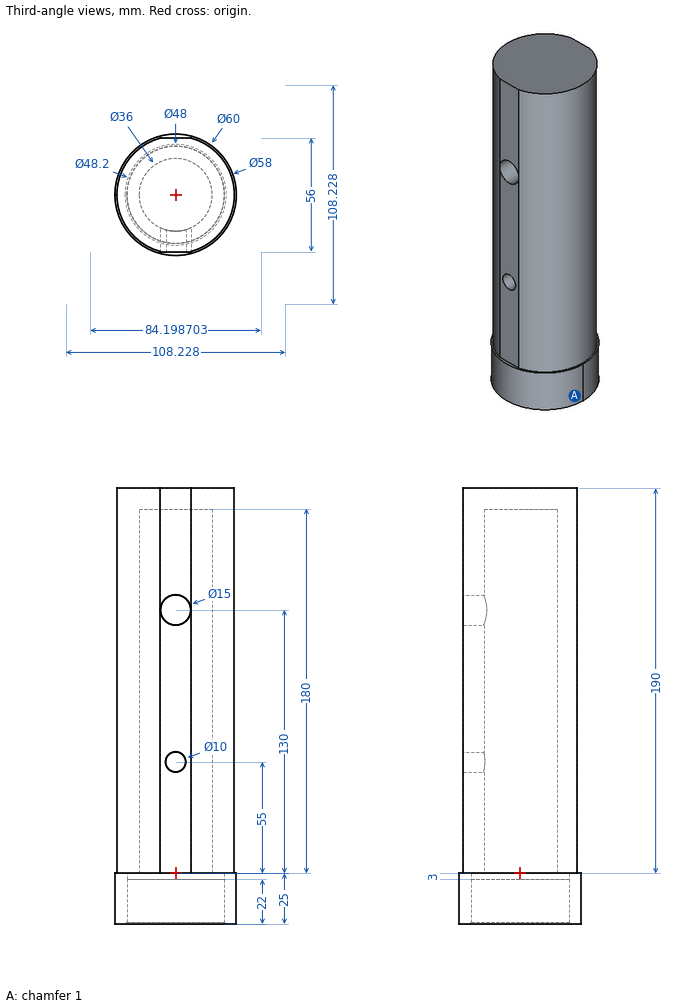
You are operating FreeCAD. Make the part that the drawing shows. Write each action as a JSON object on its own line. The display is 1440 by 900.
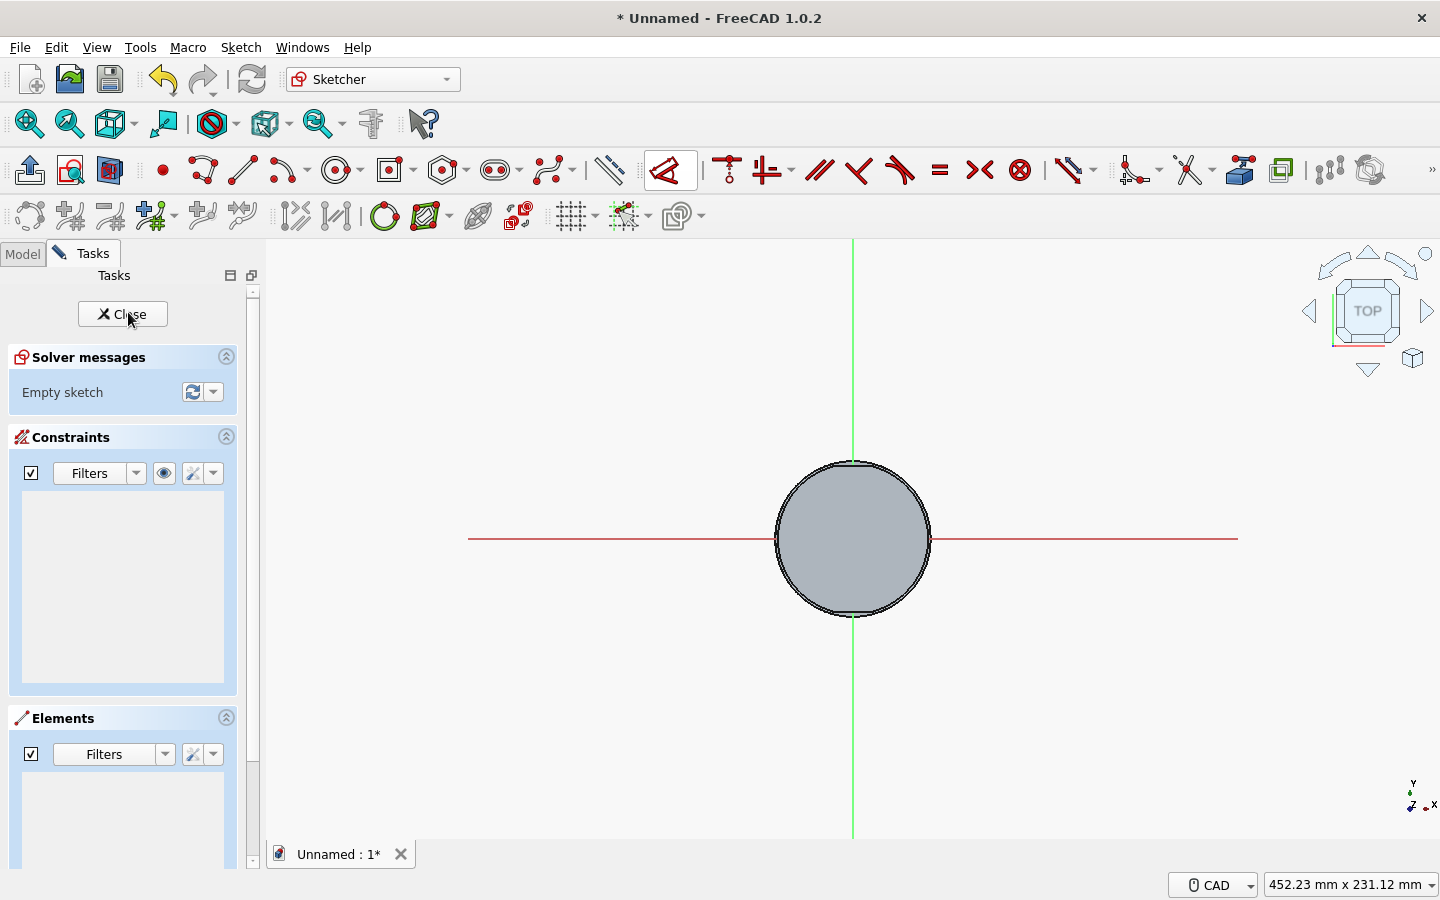
{"action": "left_click", "coordinate": [110, 170]}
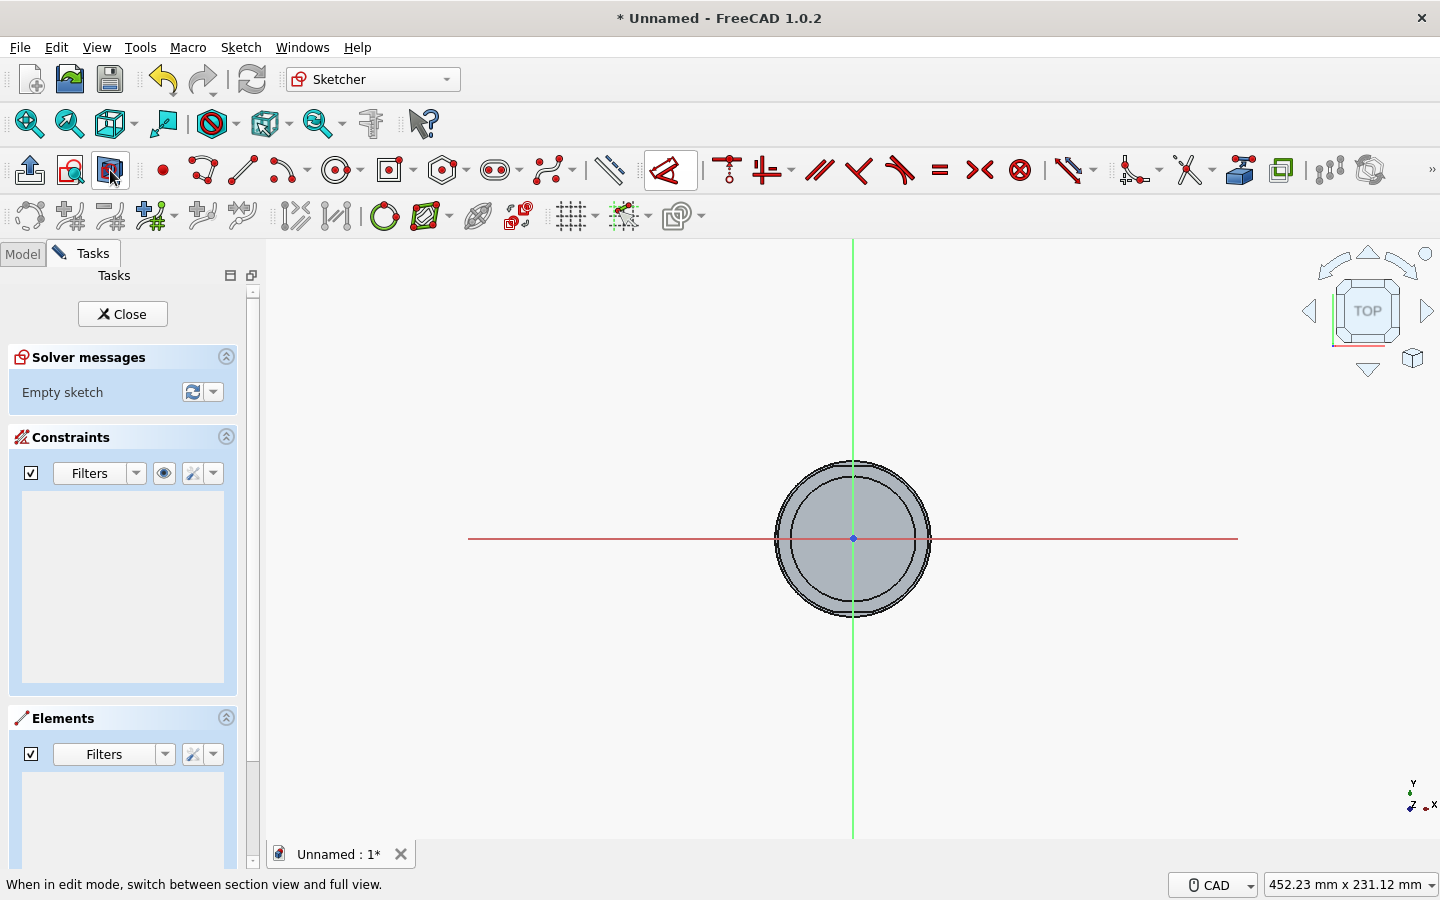
{"action": "scroll", "coordinate": [875, 539], "scroll_direction": "up", "scroll_amount": 7}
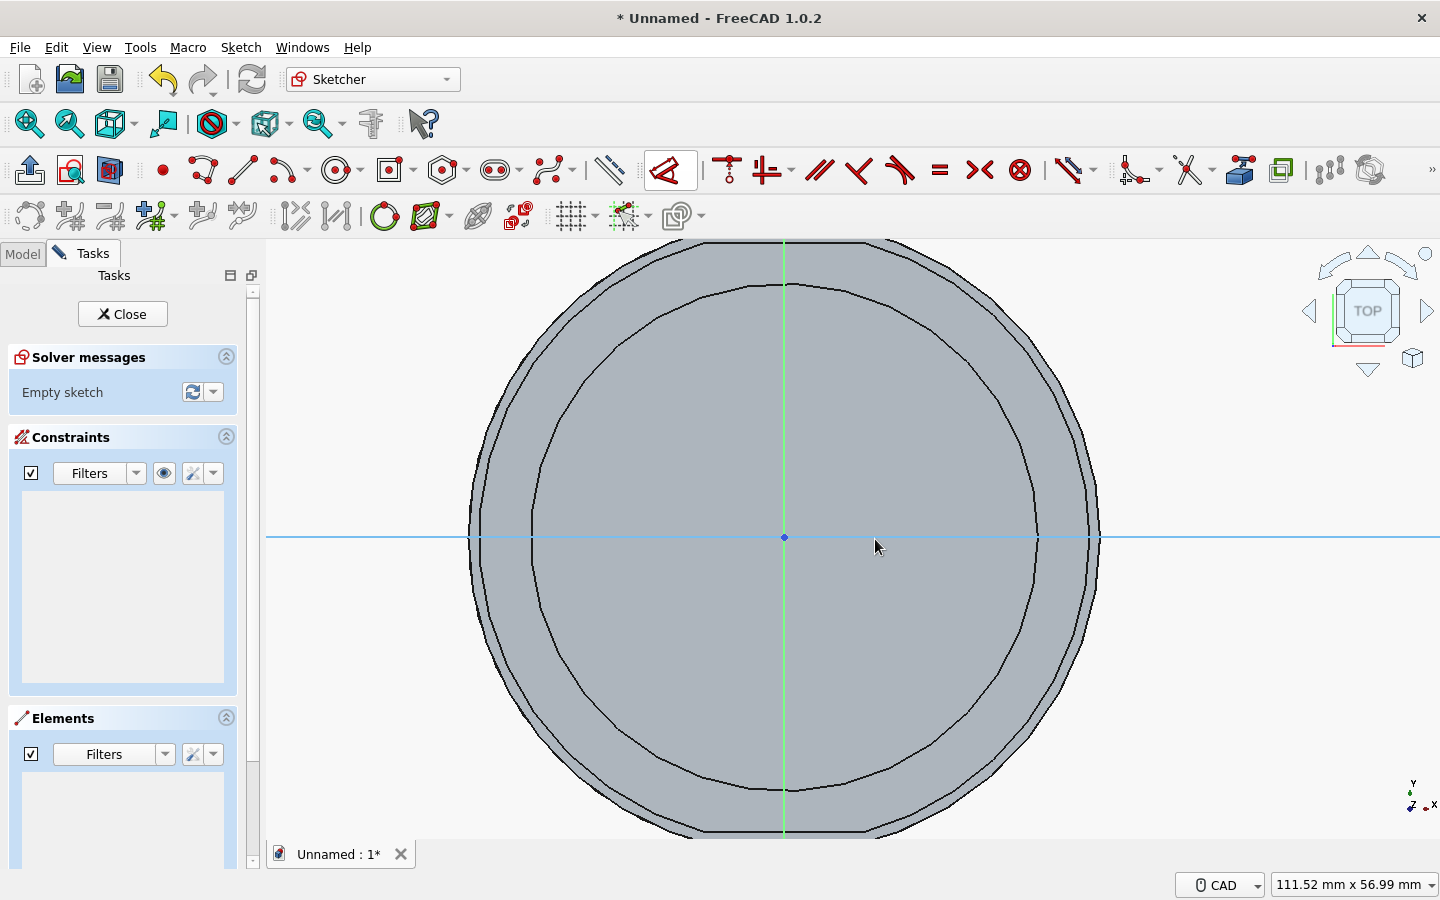
{"action": "left_click", "coordinate": [336, 170]}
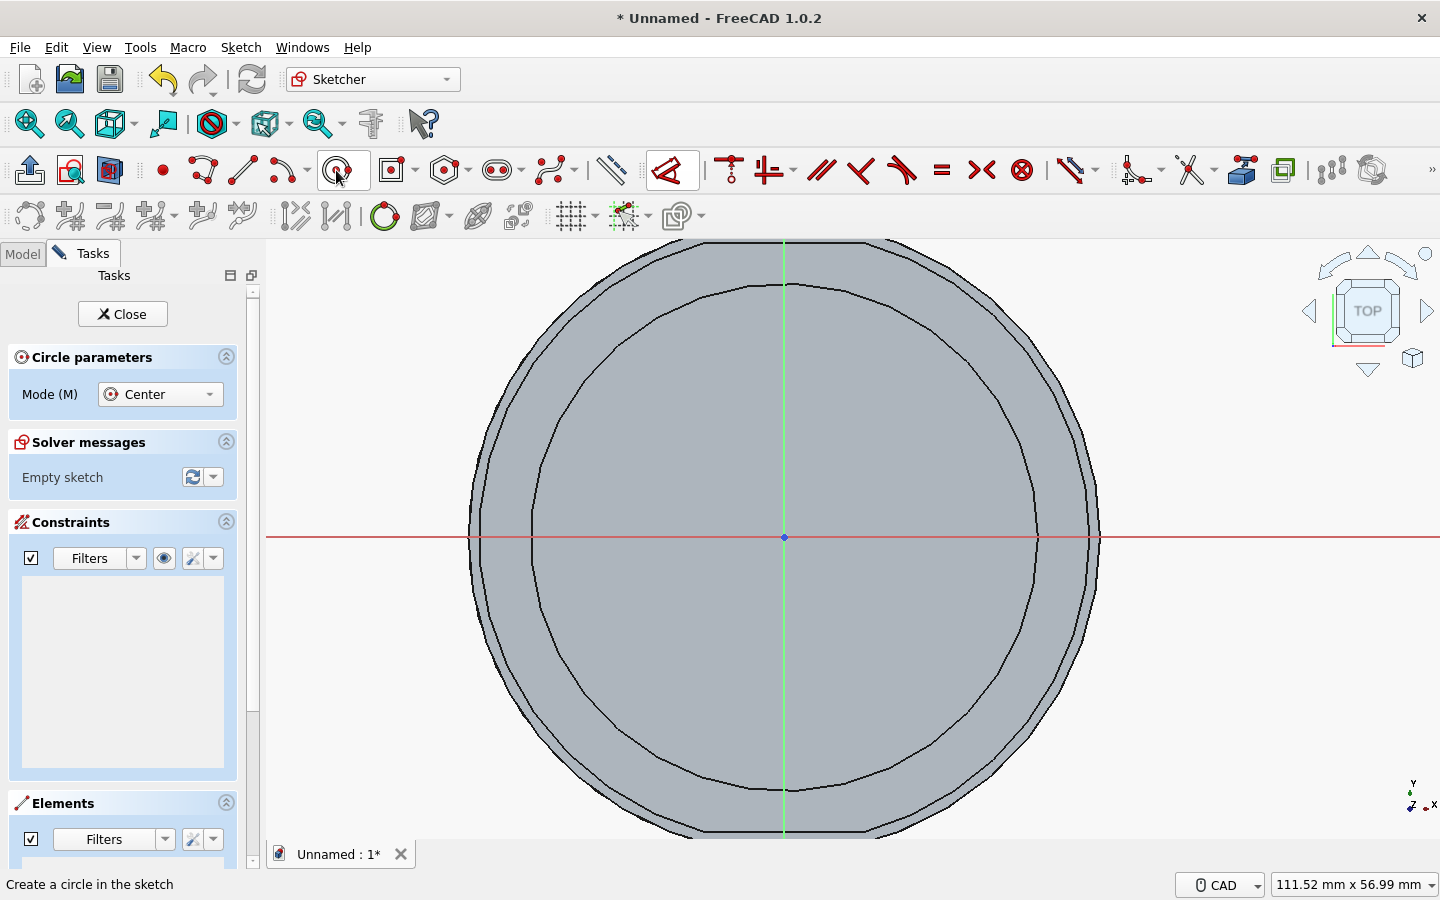
{"action": "left_click", "coordinate": [784, 537]}
{"action": "left_click", "coordinate": [918, 403]}
{"action": "key", "text": "Escape"}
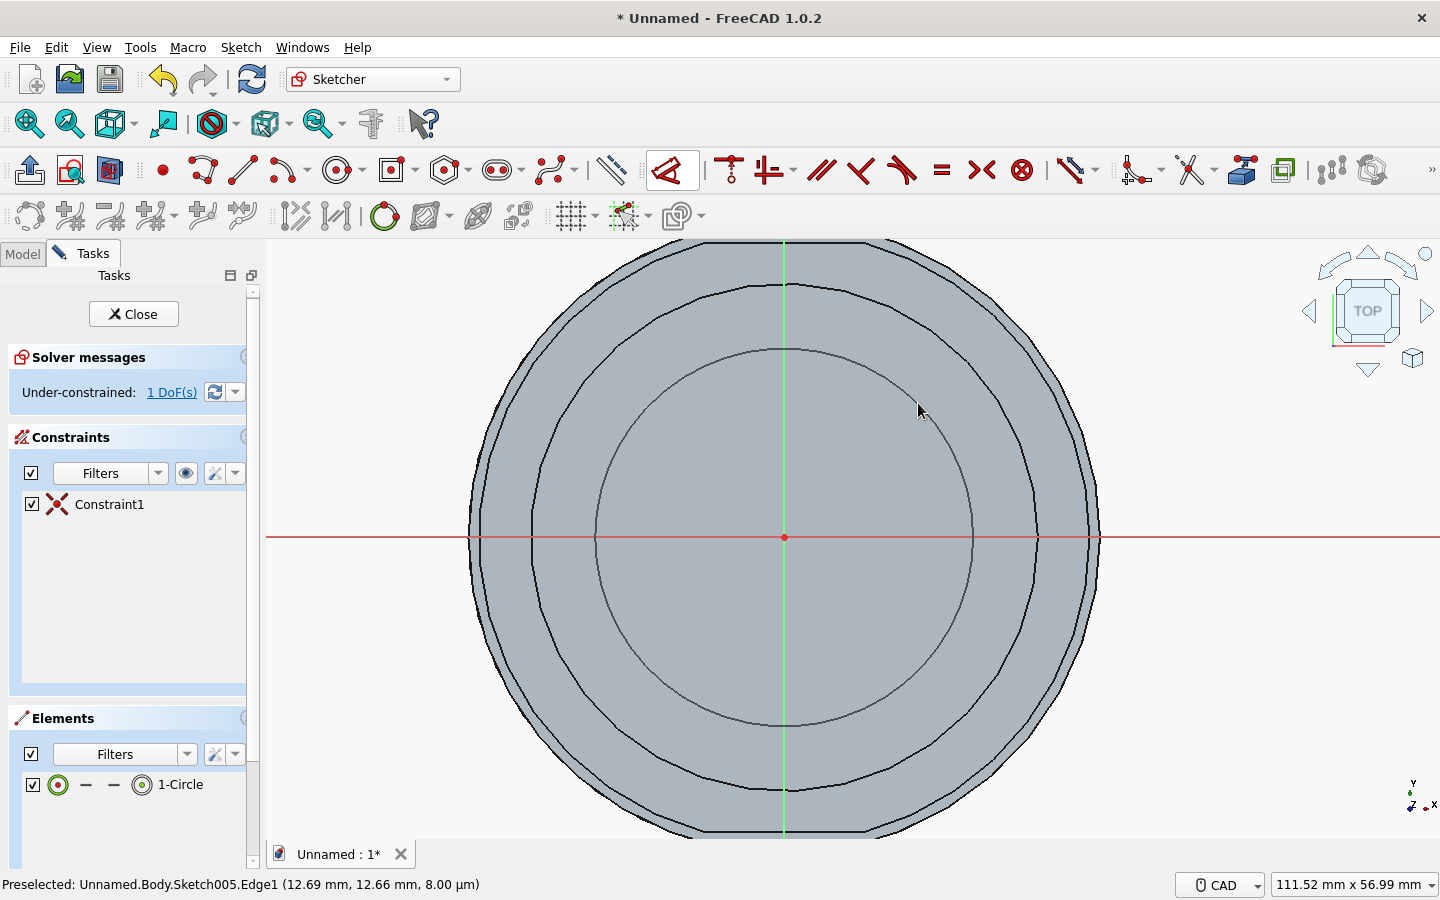
{"action": "left_click", "coordinate": [917, 403]}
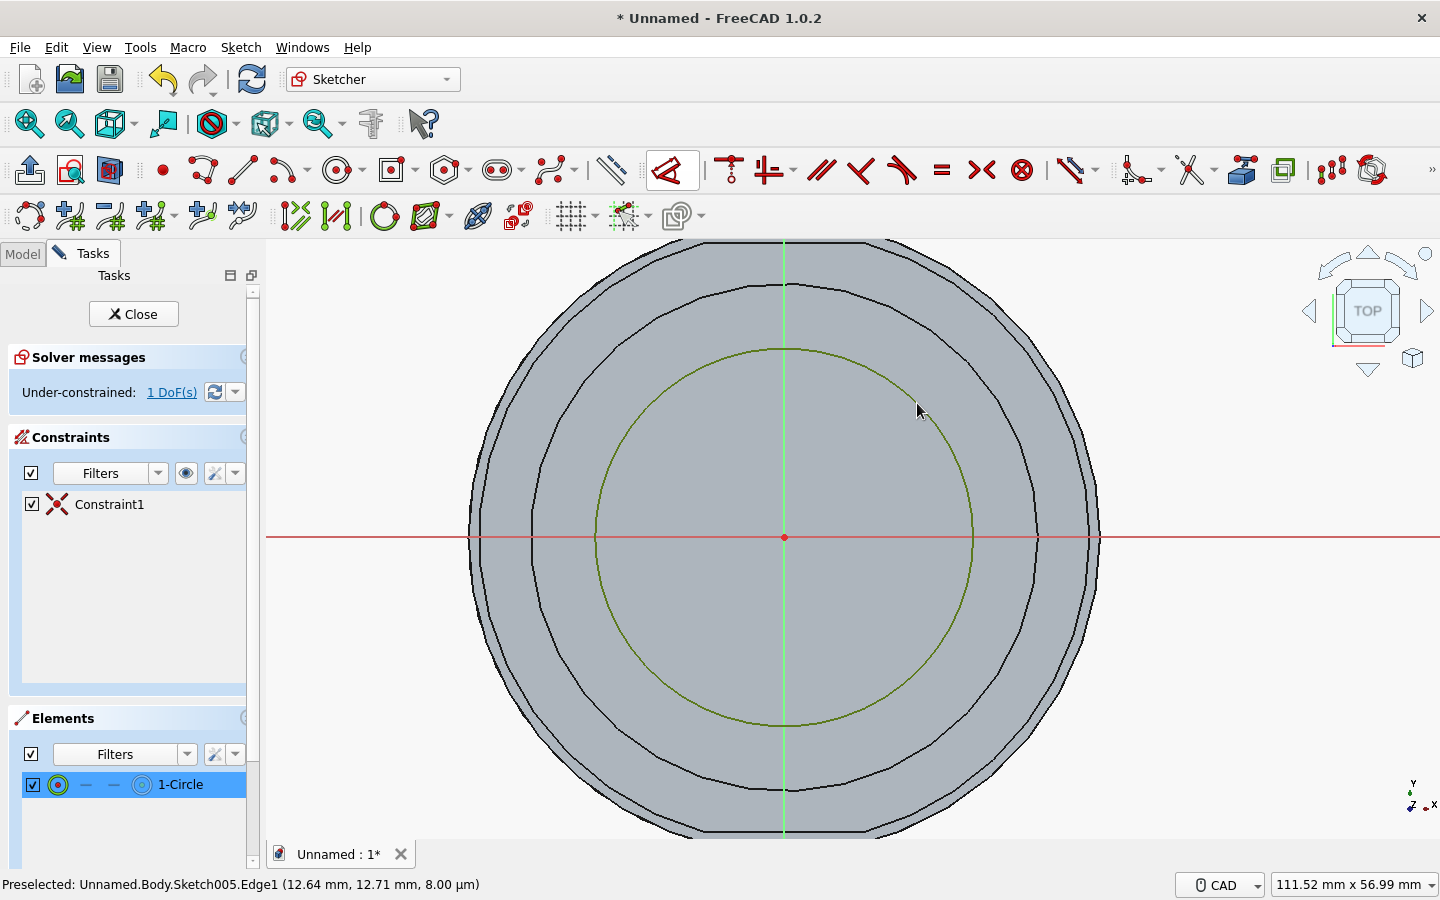
{"action": "key", "text": "k o"}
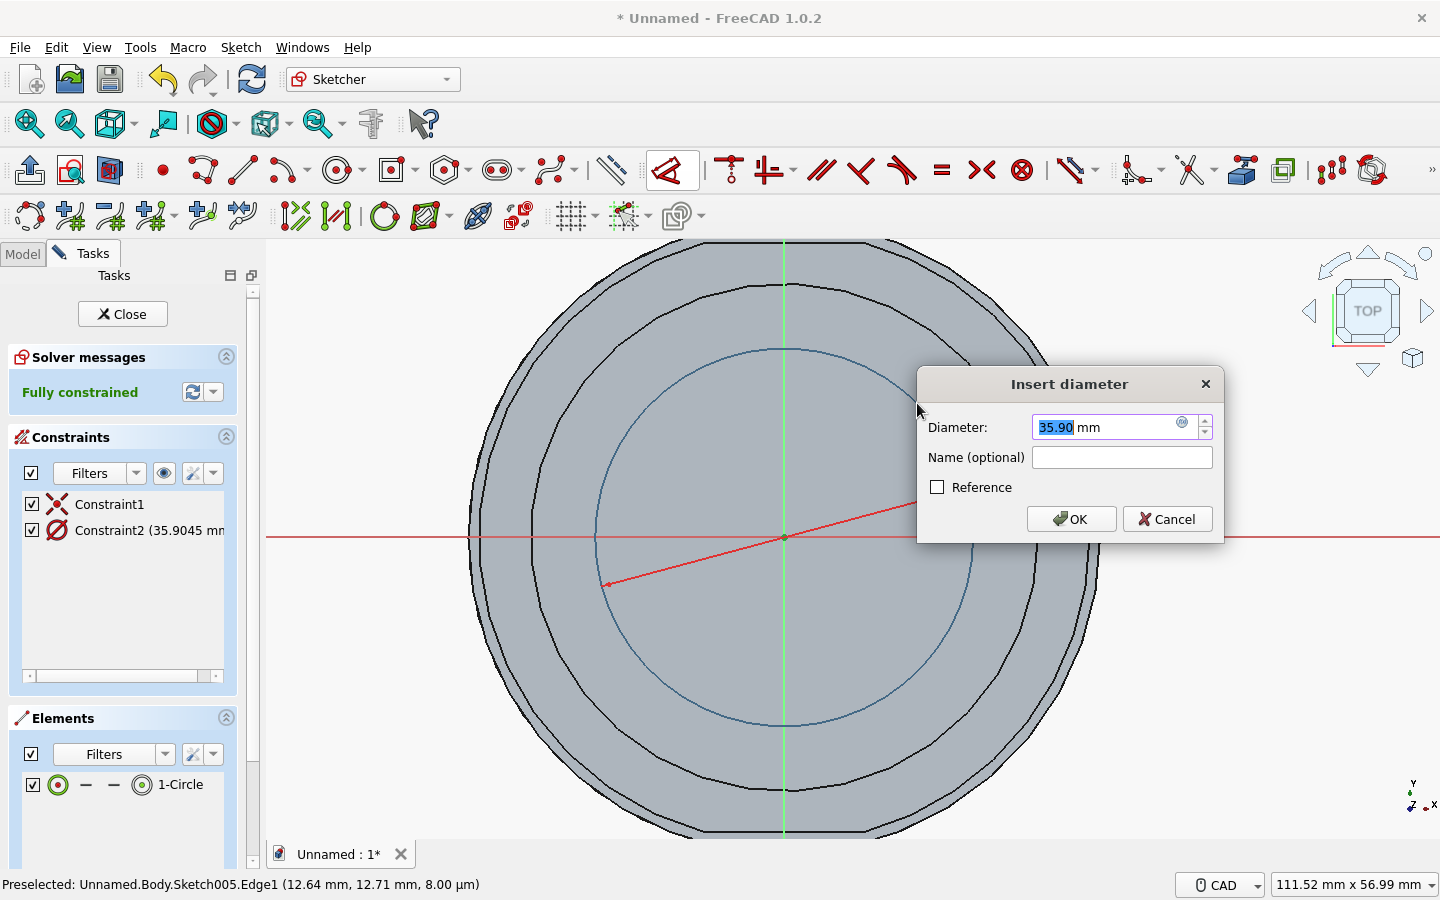
{"action": "type", "text": "36"}
{"action": "key", "text": "Return"}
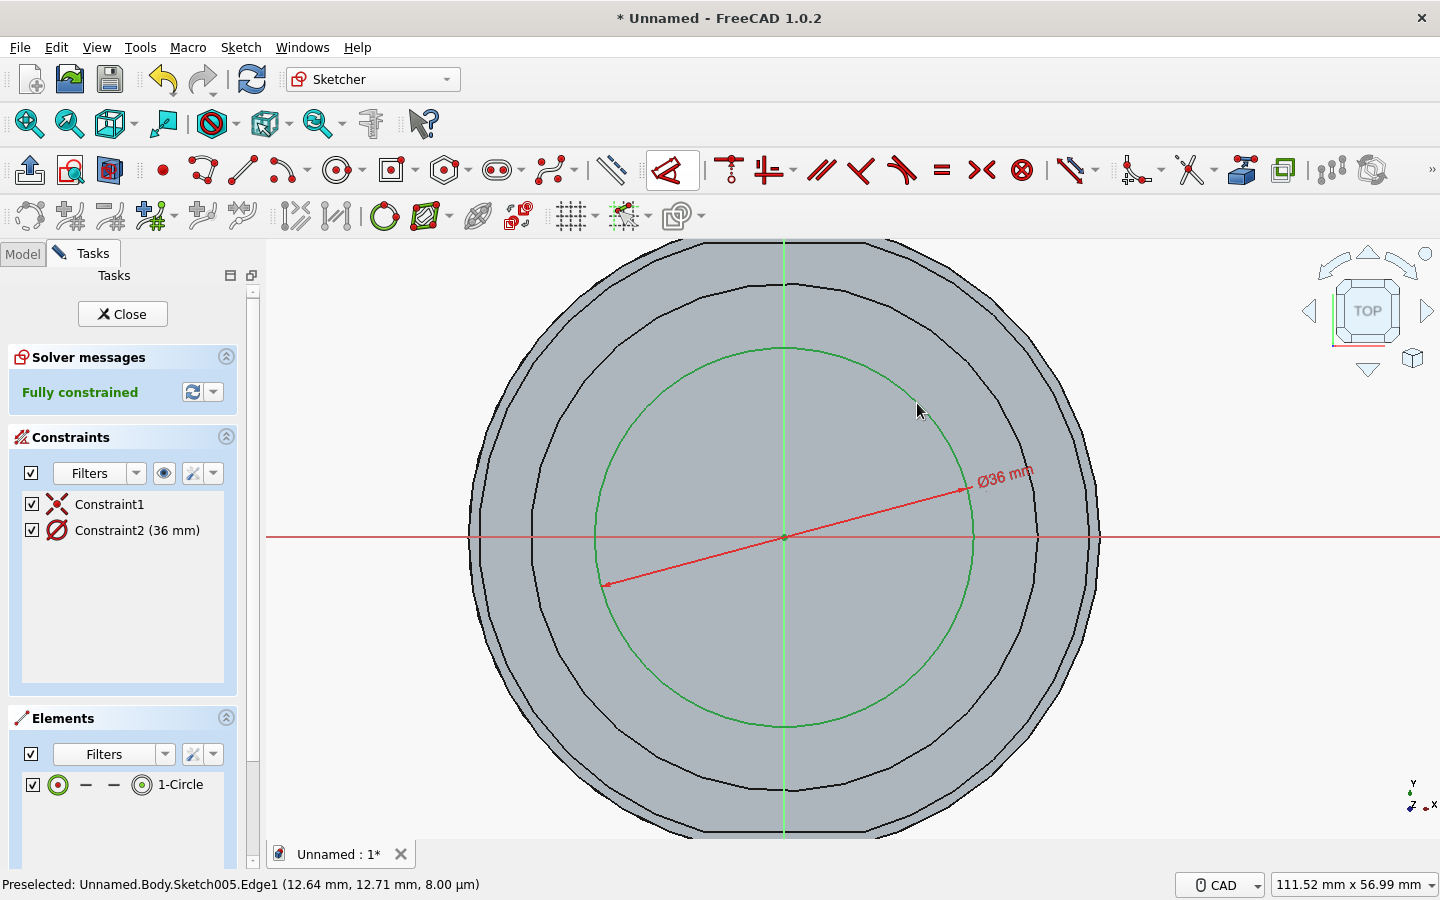
{"action": "left_click", "coordinate": [123, 314]}